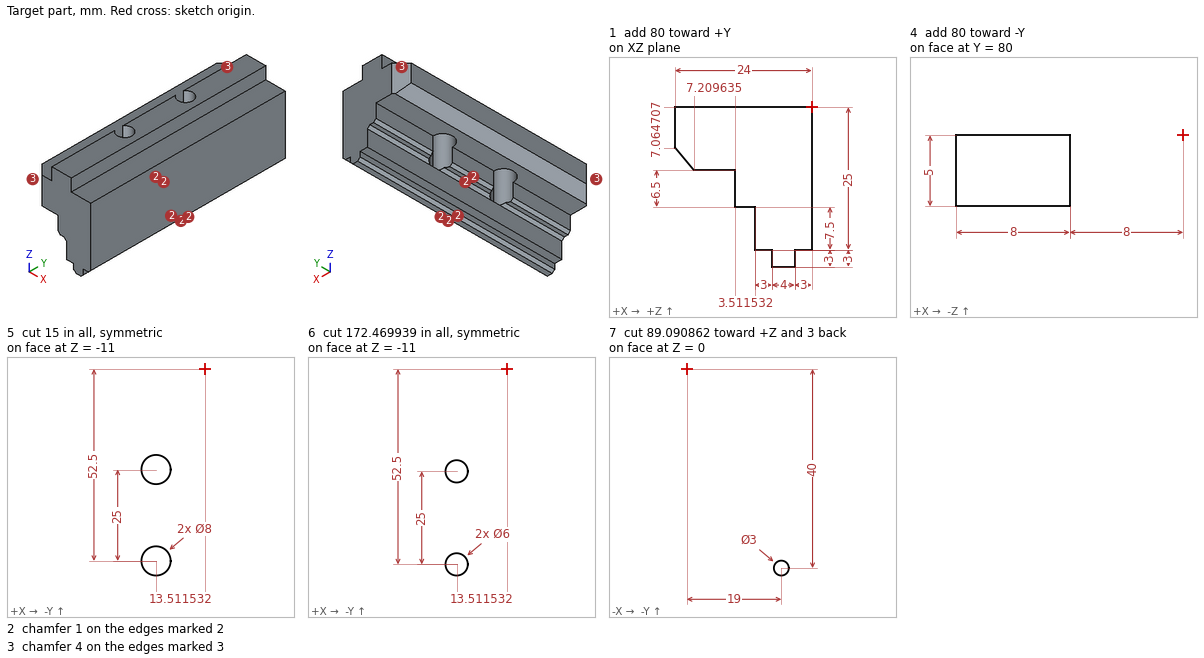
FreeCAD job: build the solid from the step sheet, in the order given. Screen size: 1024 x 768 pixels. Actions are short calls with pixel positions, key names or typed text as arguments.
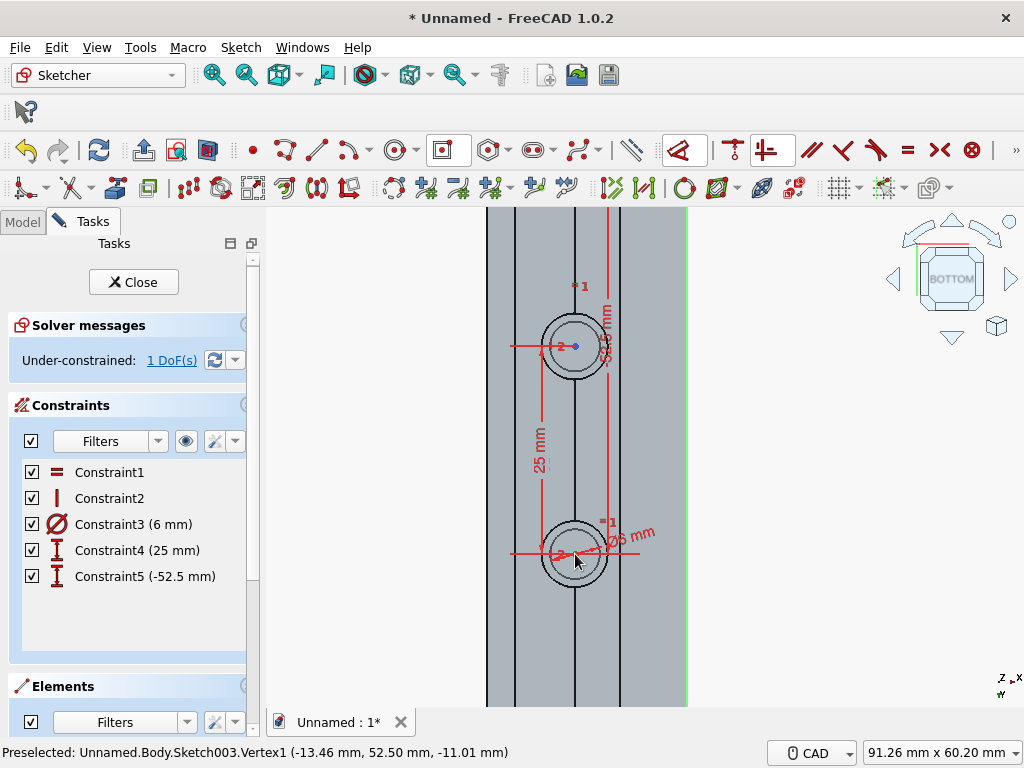
click(702, 150)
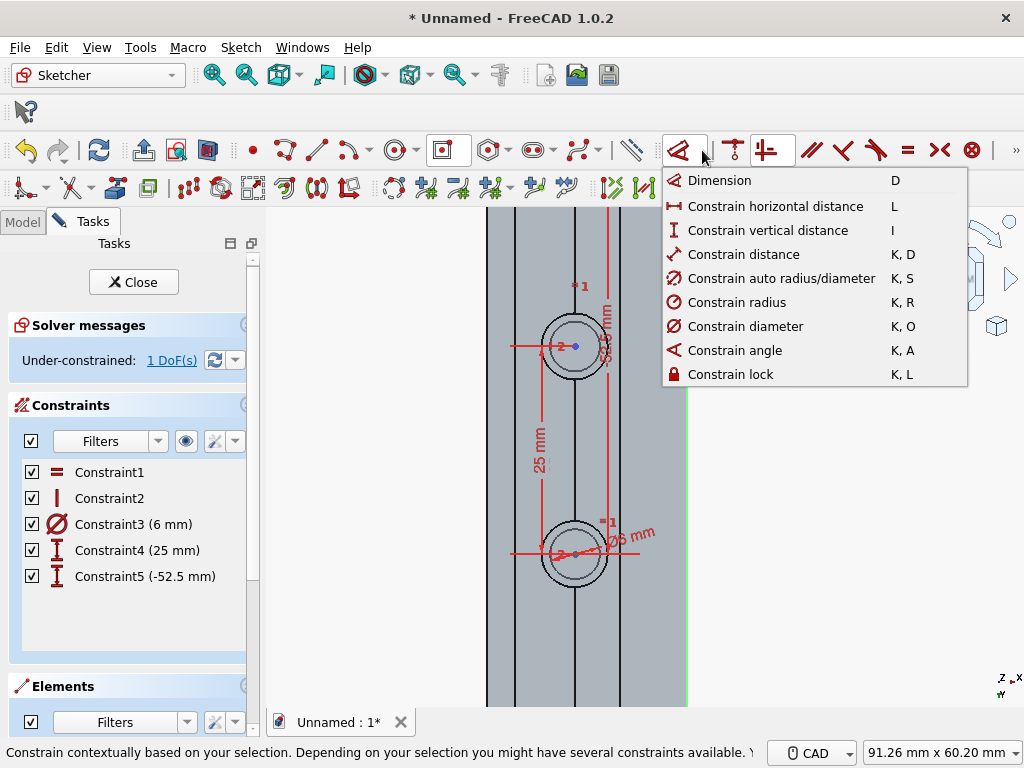
click(815, 206)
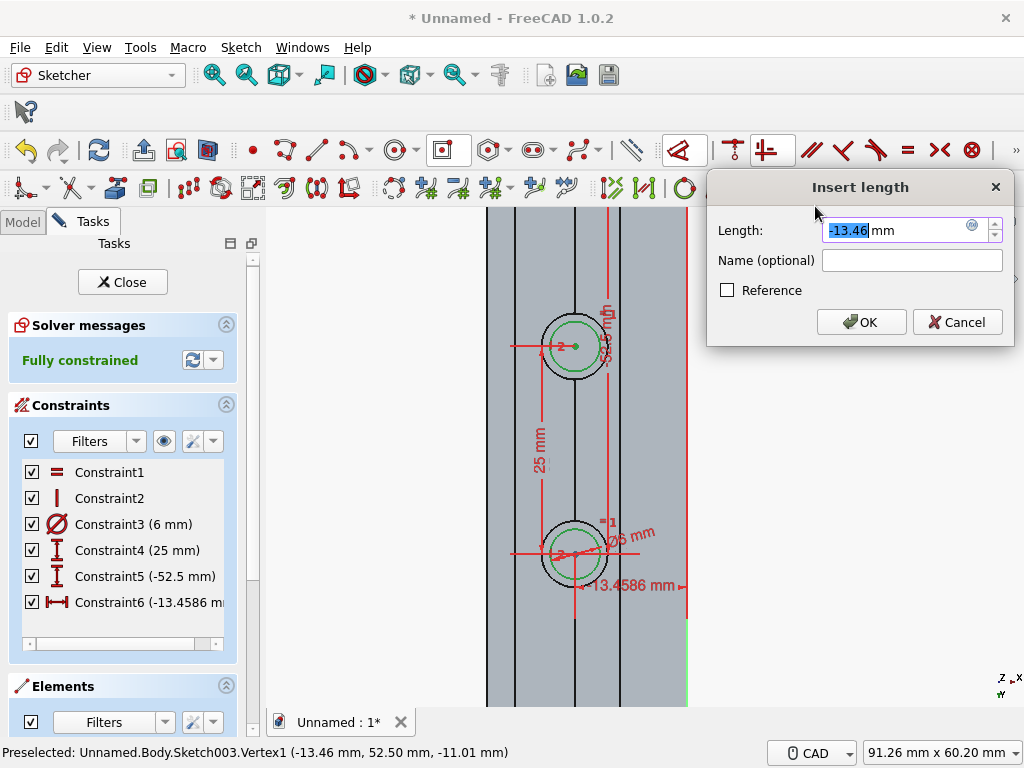
text(-13.511532)
key(Return)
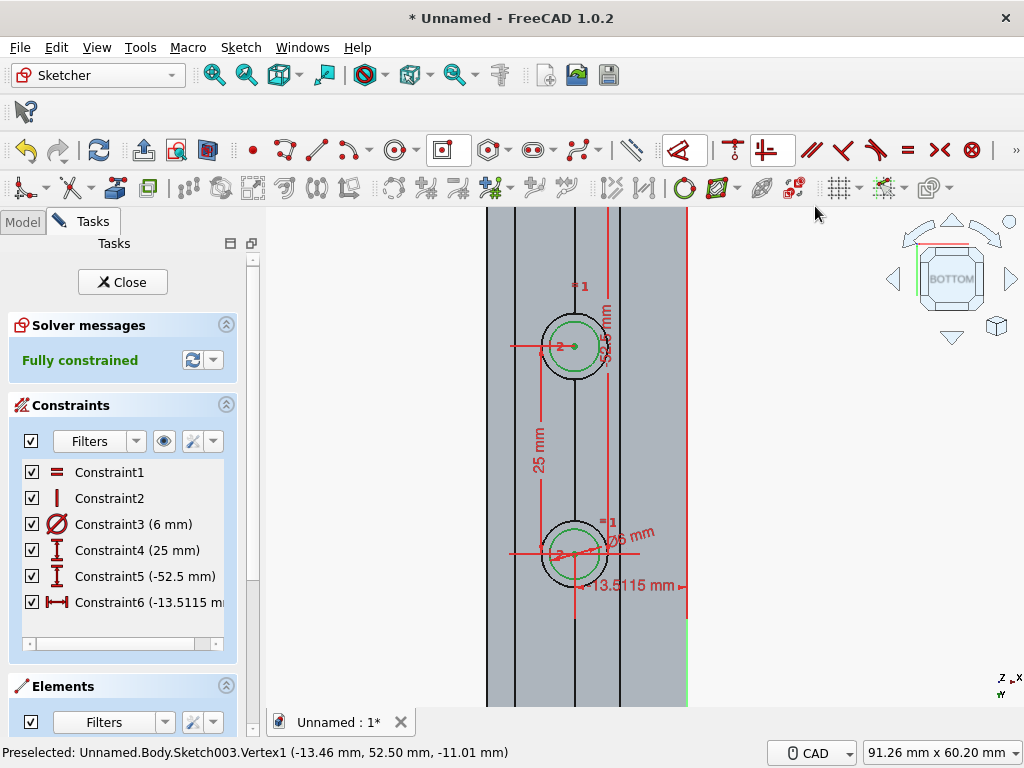
click(123, 282)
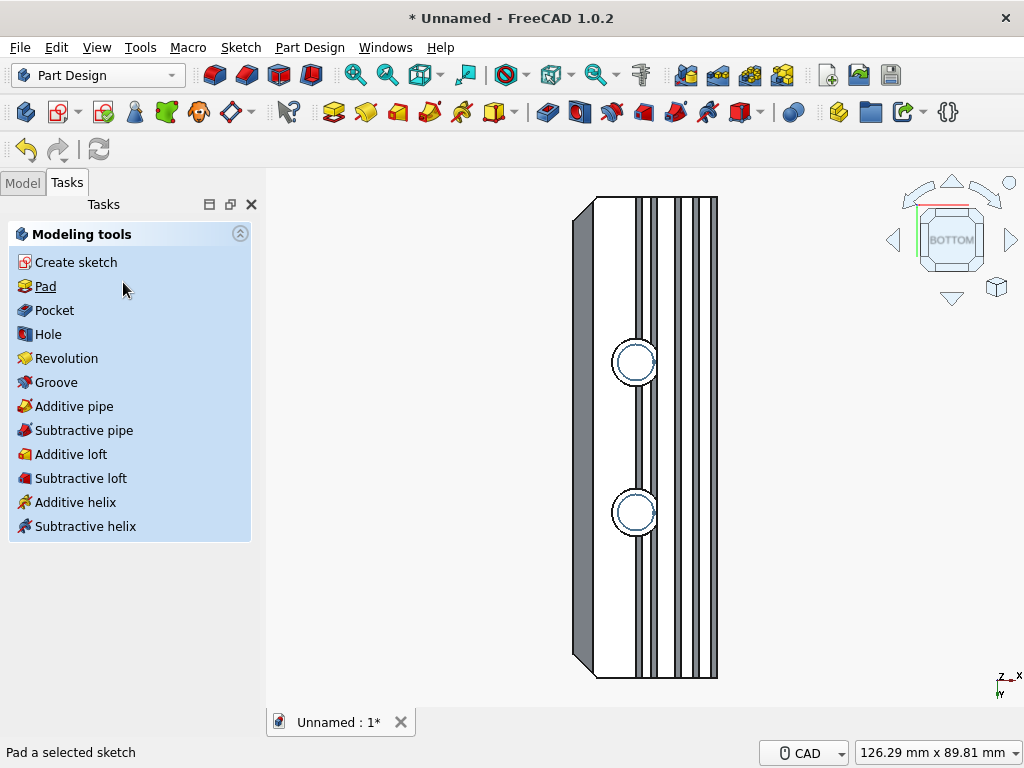
click(548, 112)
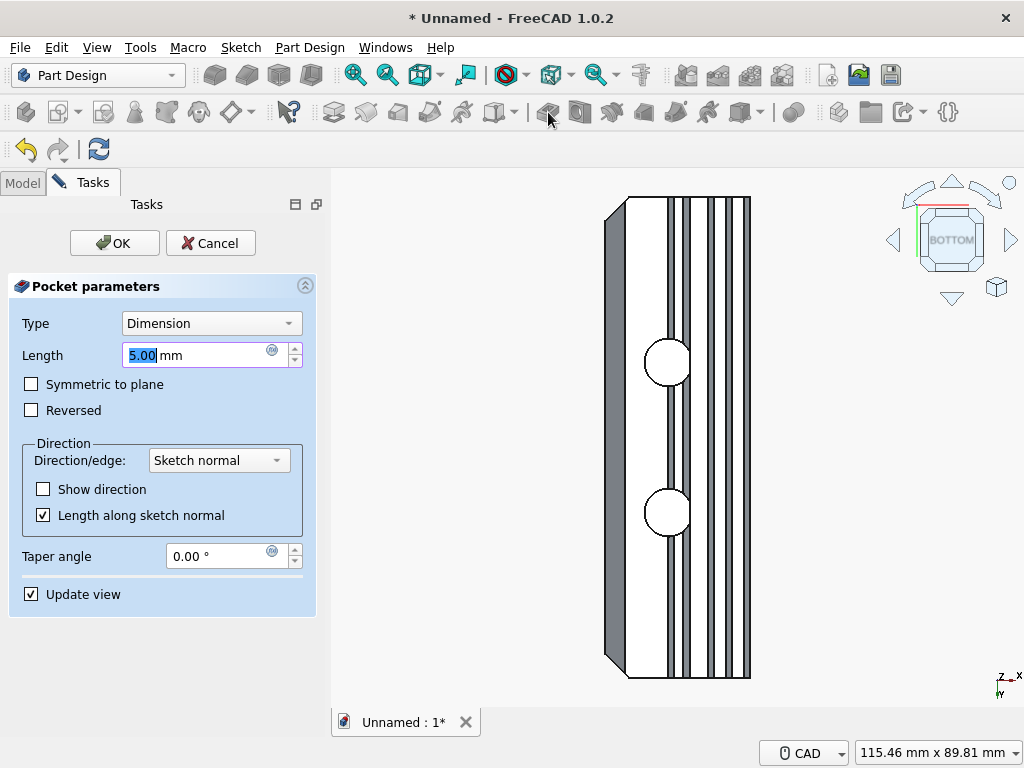
text(172.469939)
key(Tab)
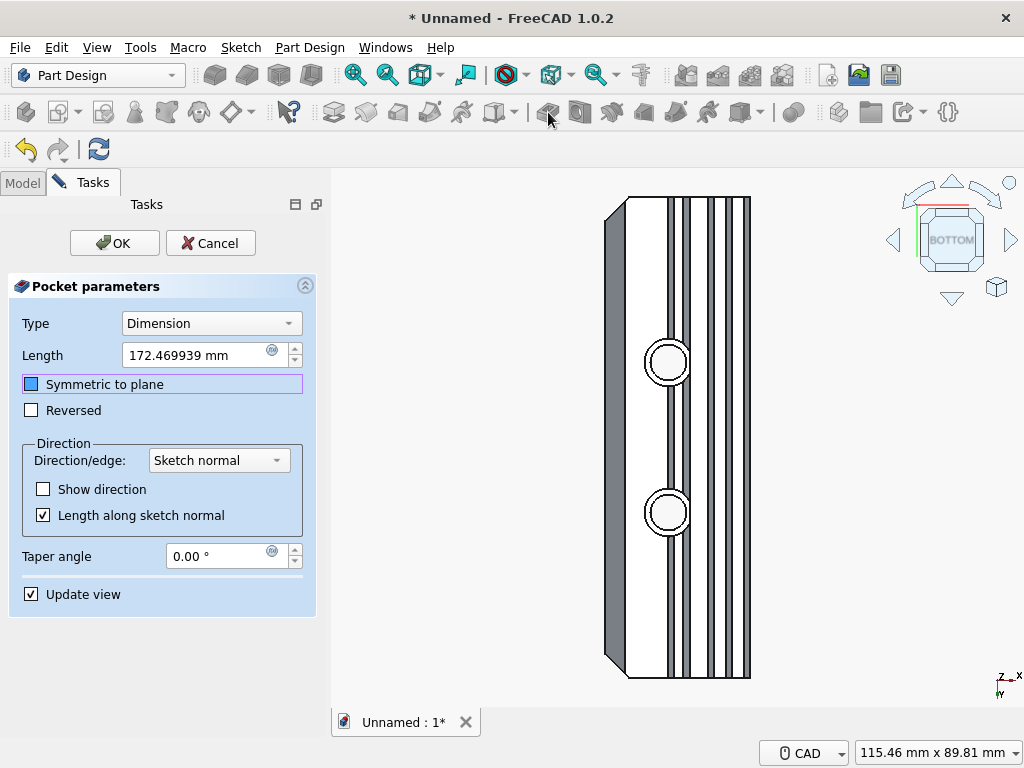
click(30, 384)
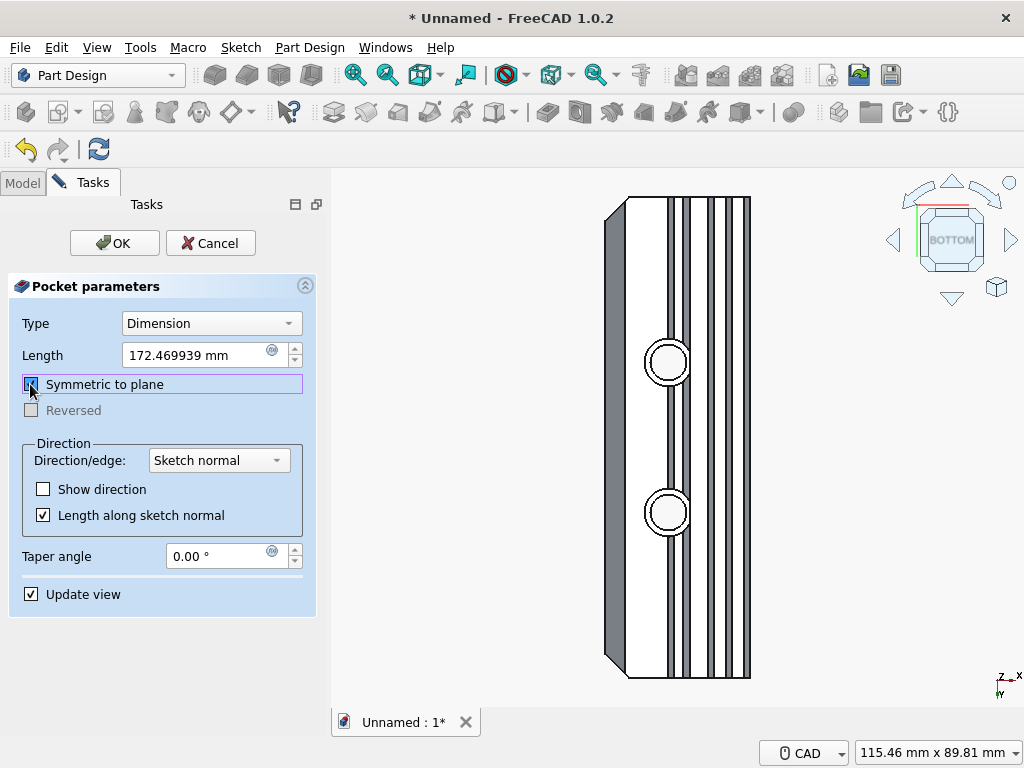
click(115, 243)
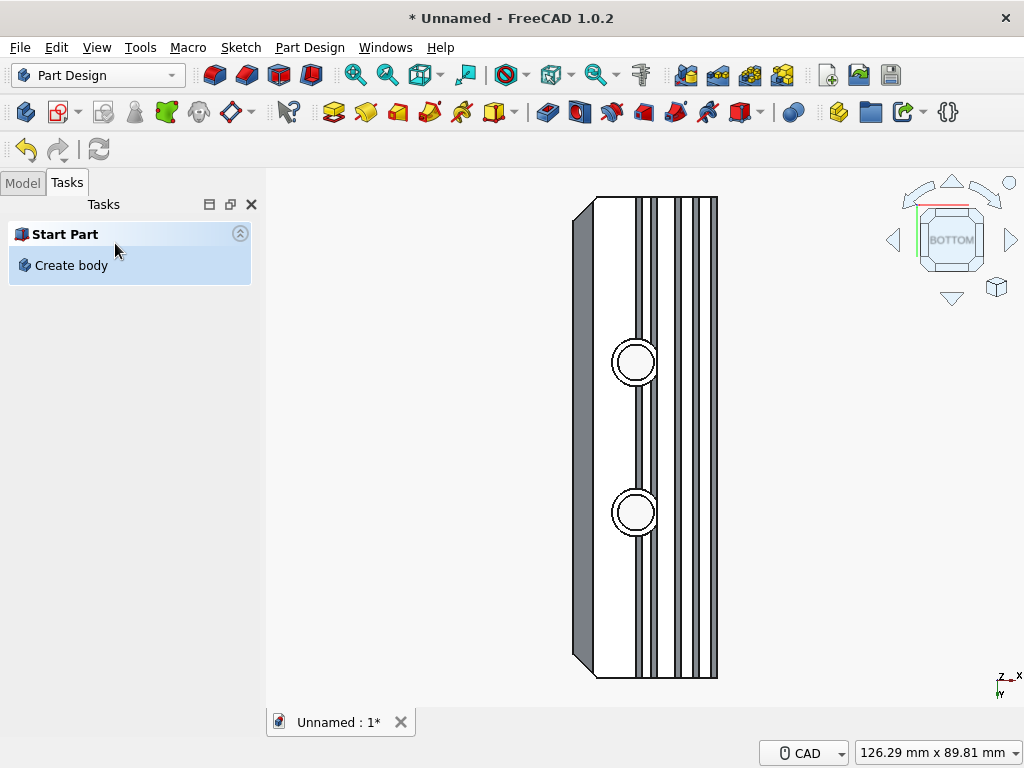
key(0)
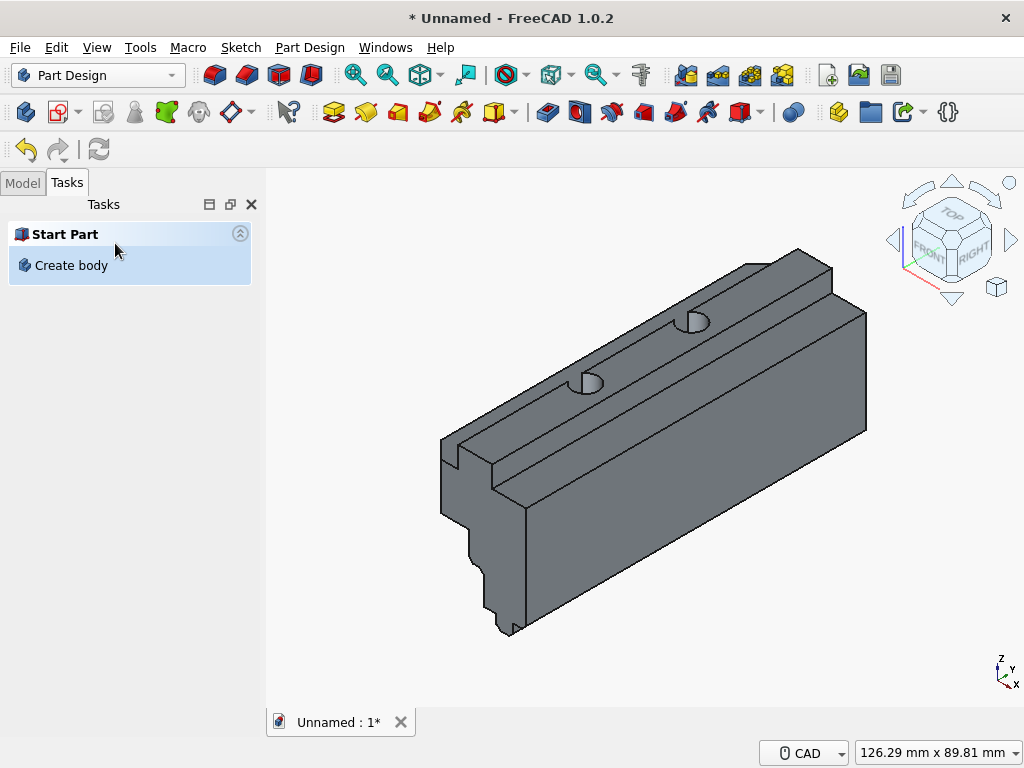
click(824, 316)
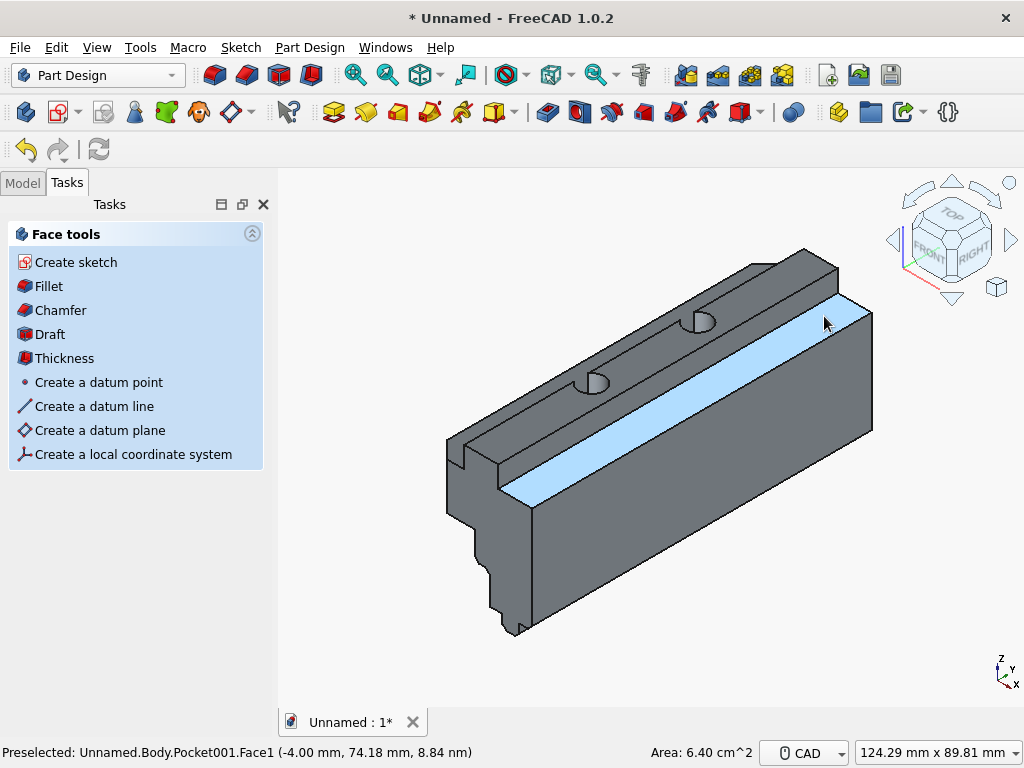
click(58, 112)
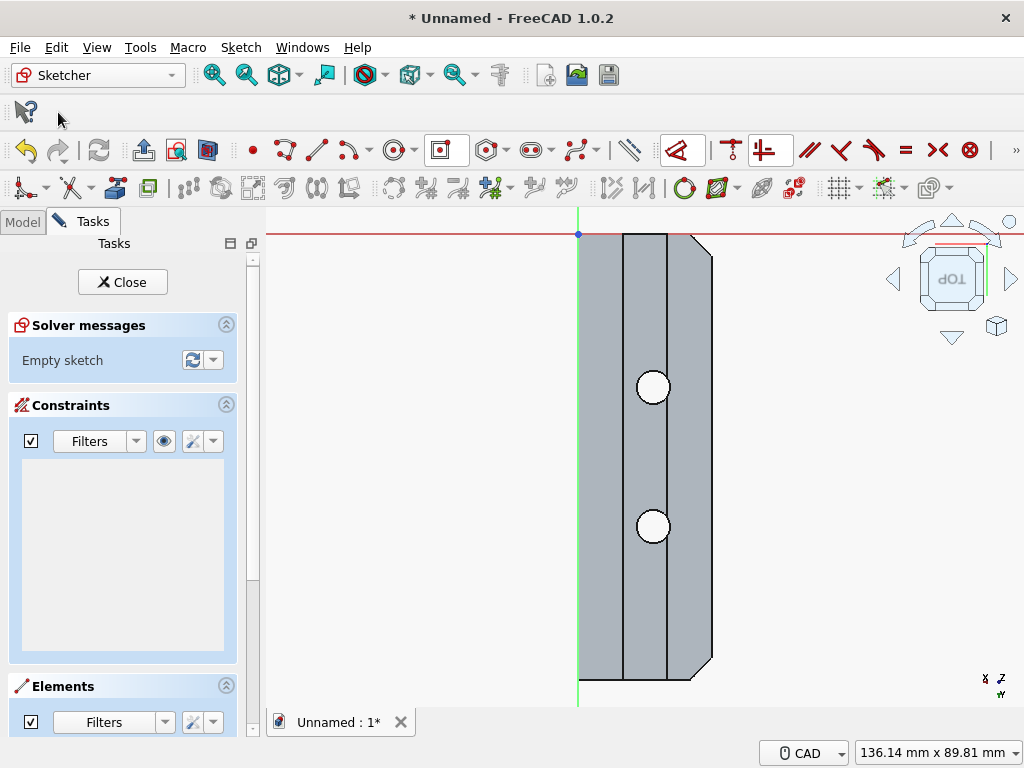
key(q)
key(s)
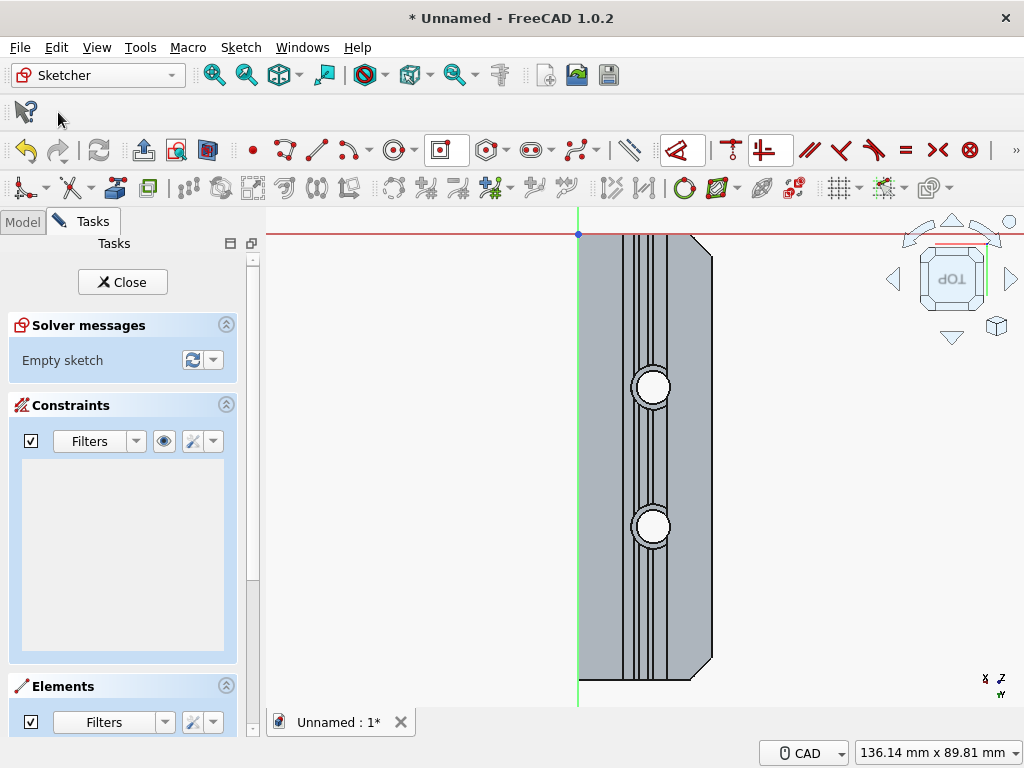
scroll(690, 457, up, 15)